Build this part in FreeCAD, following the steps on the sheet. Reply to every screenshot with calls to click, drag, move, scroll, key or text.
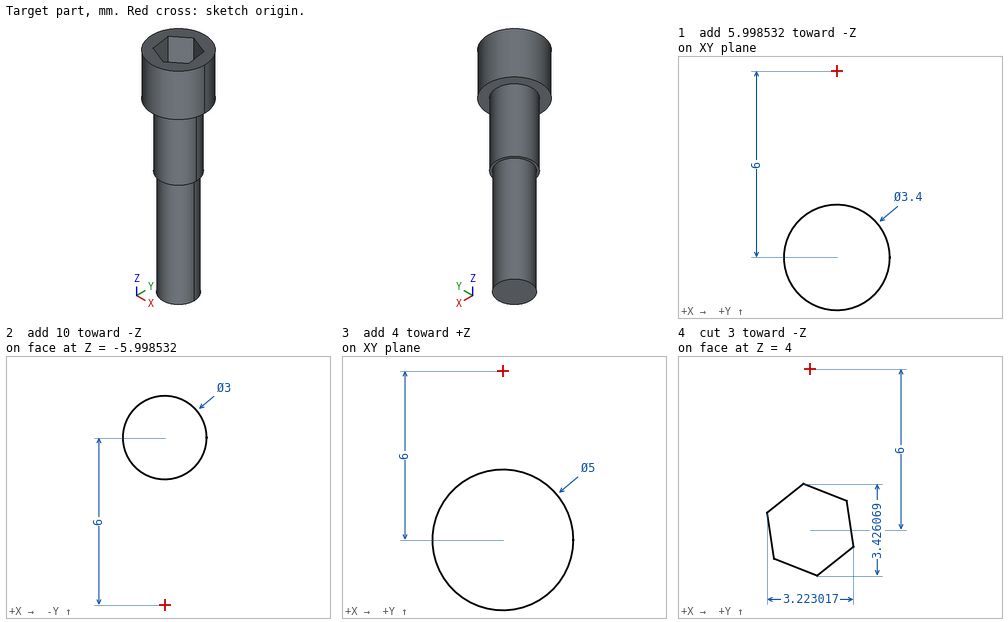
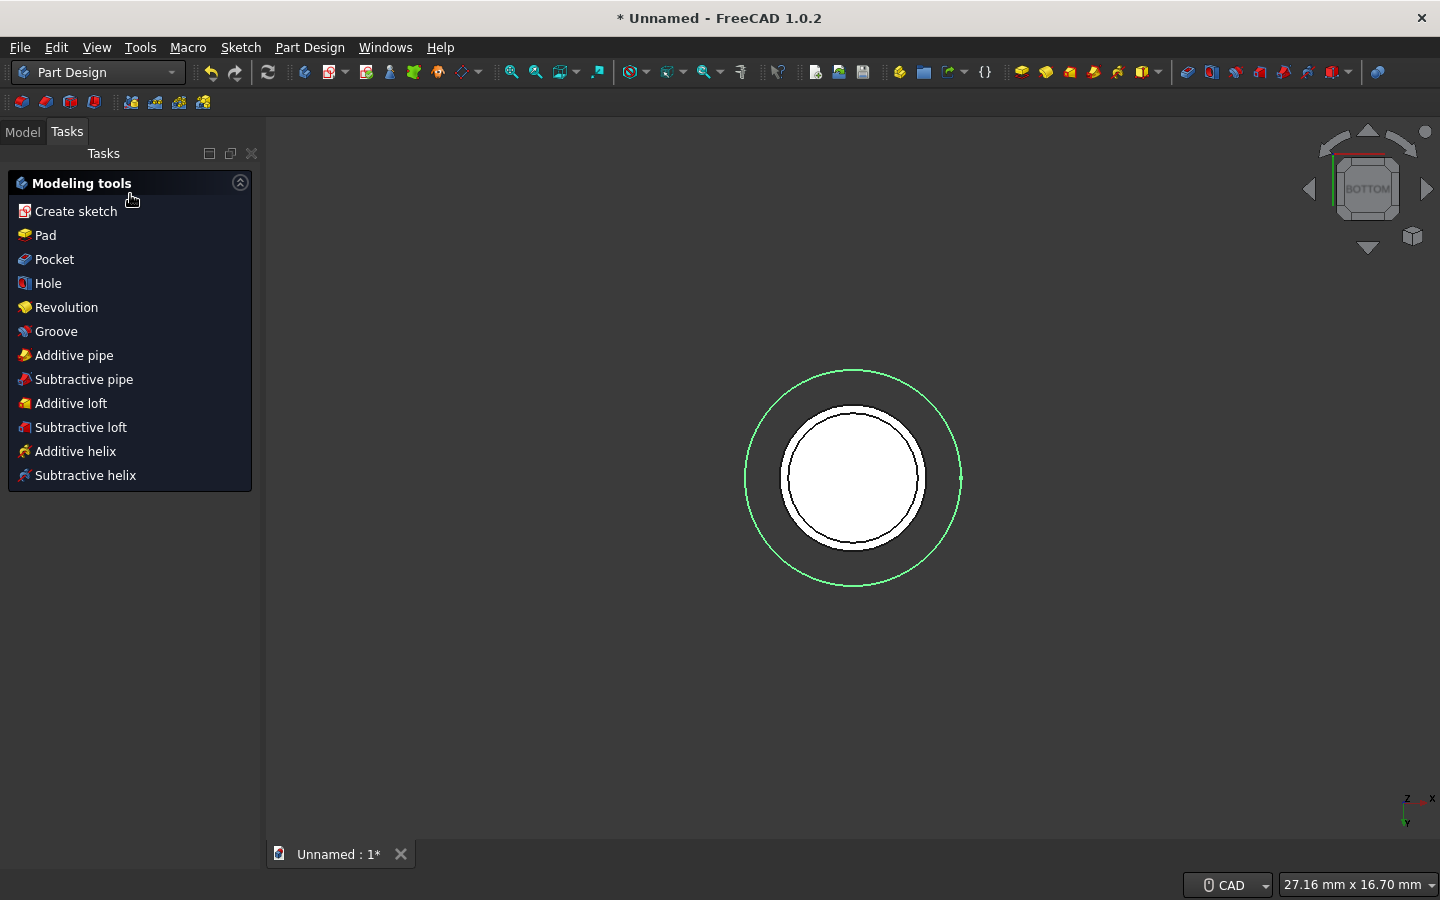
click(1022, 72)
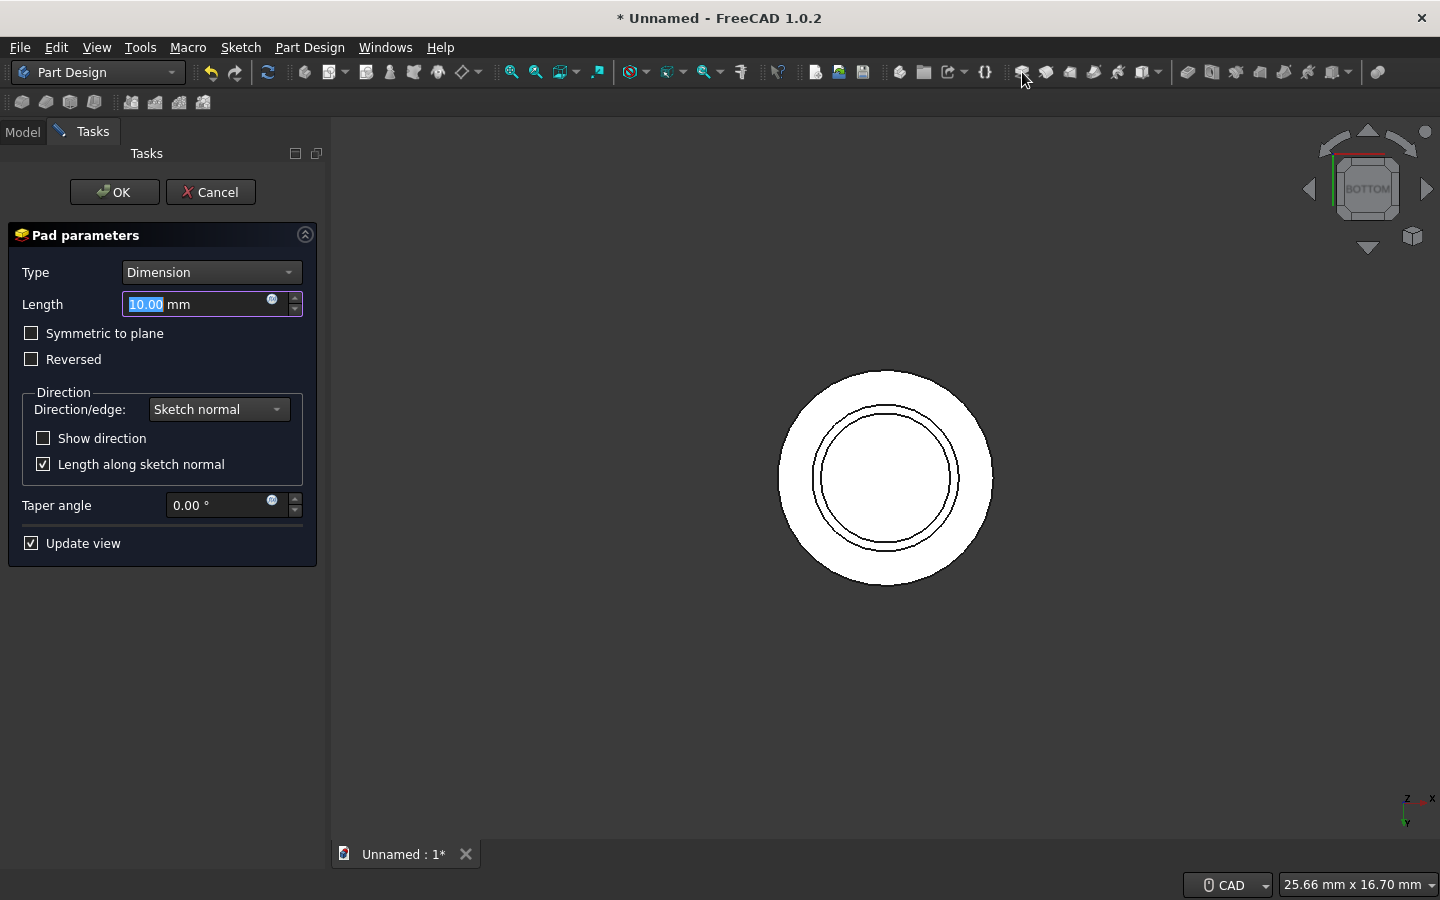
text(4)
key(Tab)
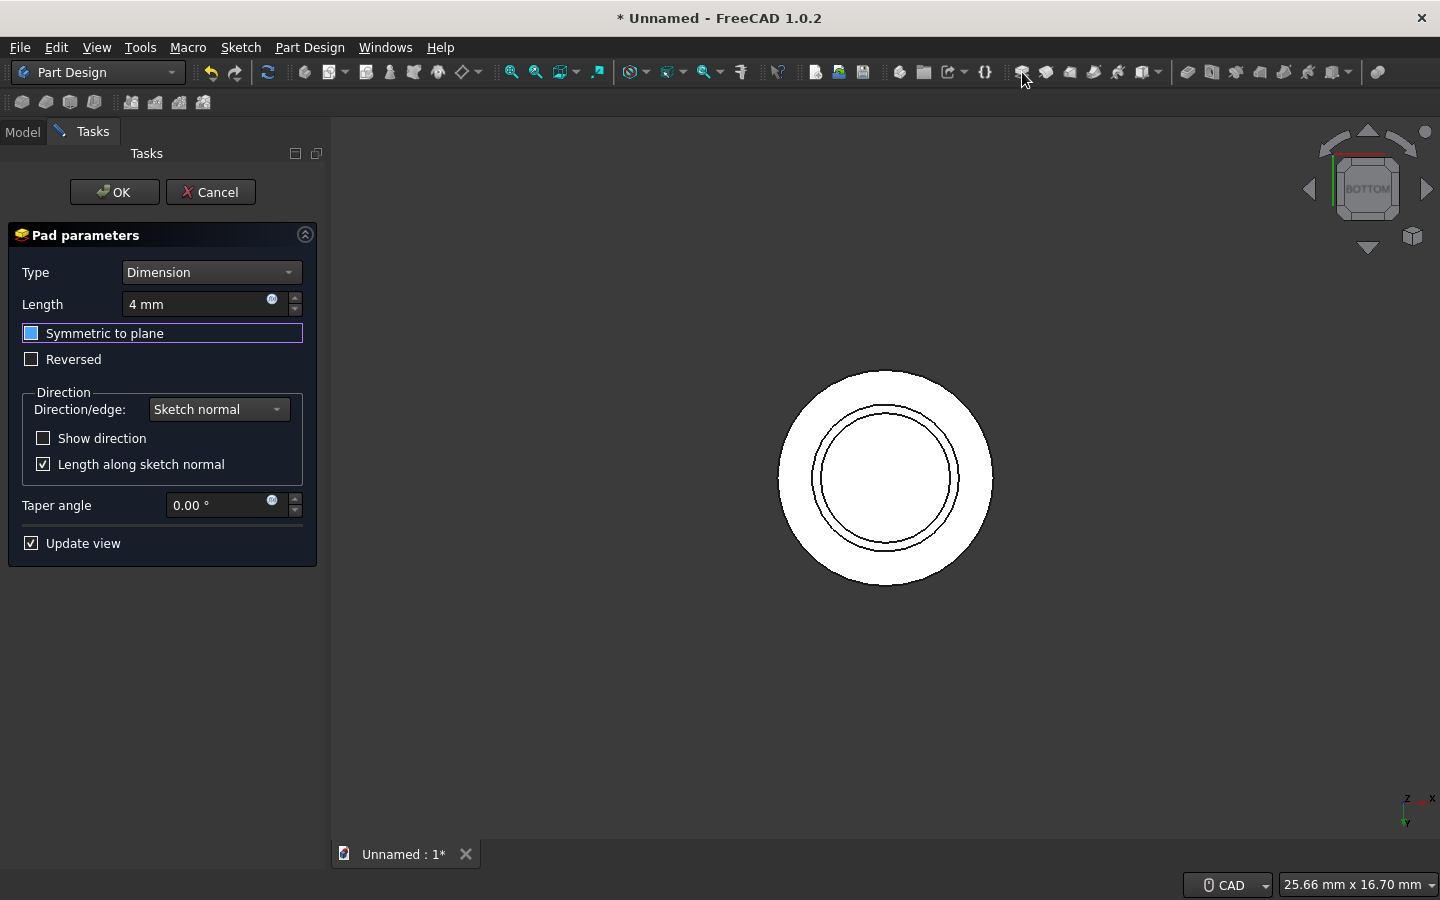
click(115, 192)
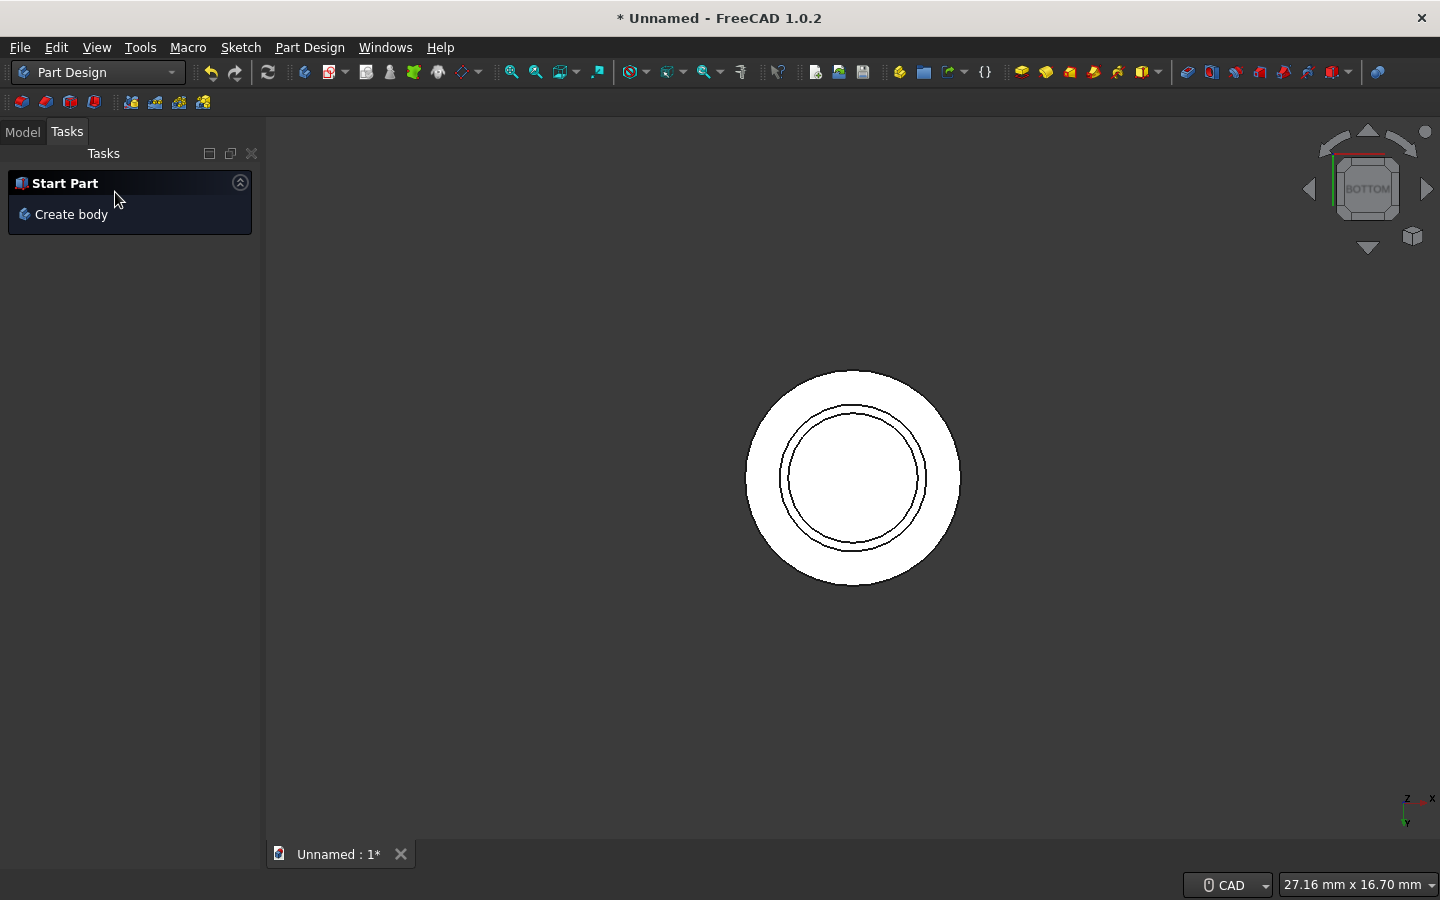
key(v)
key(f)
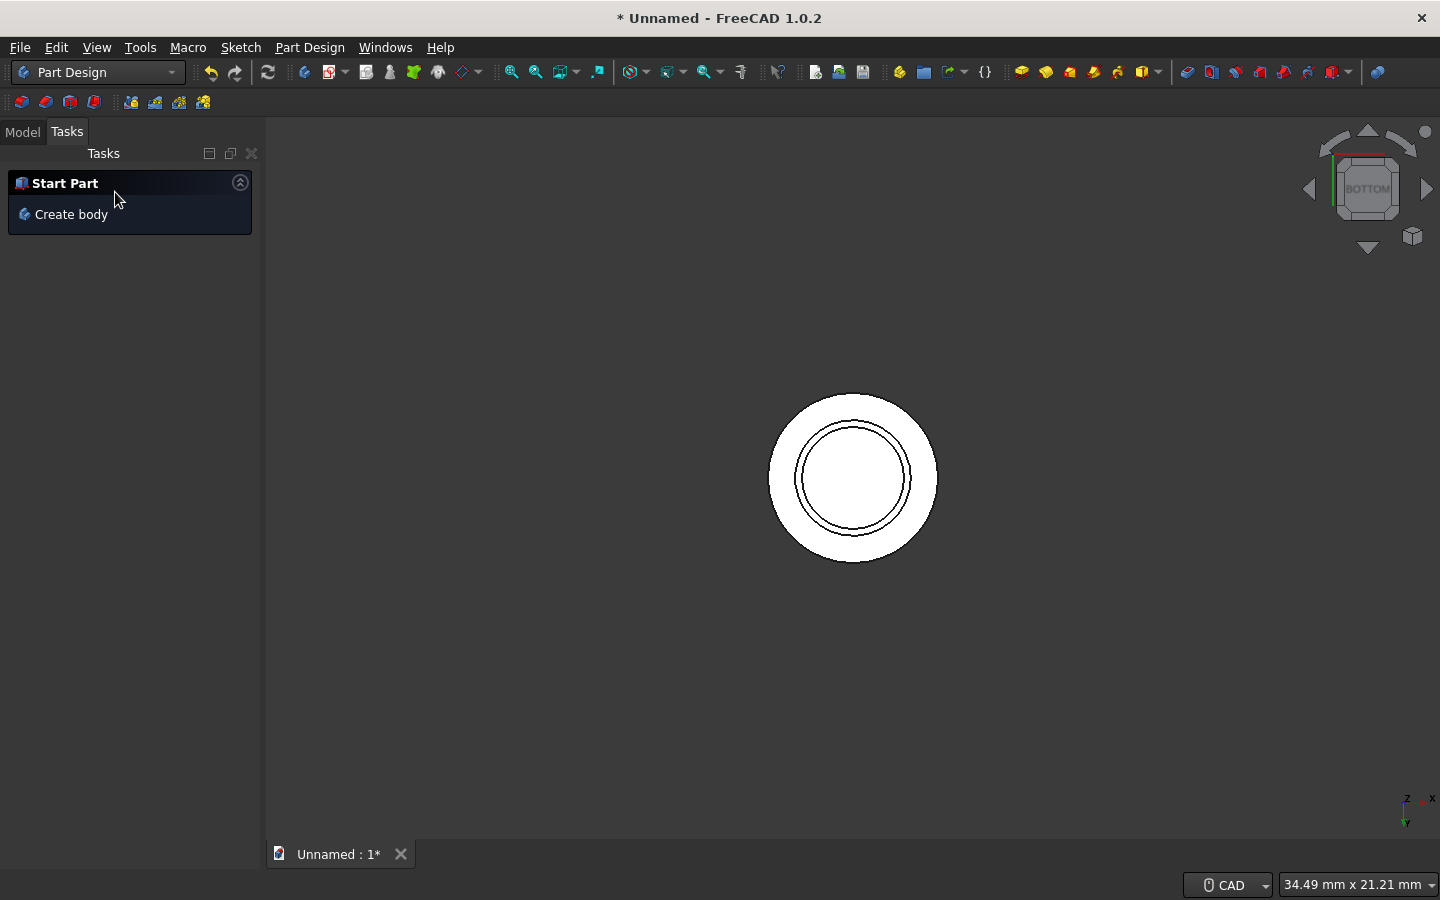
key(0)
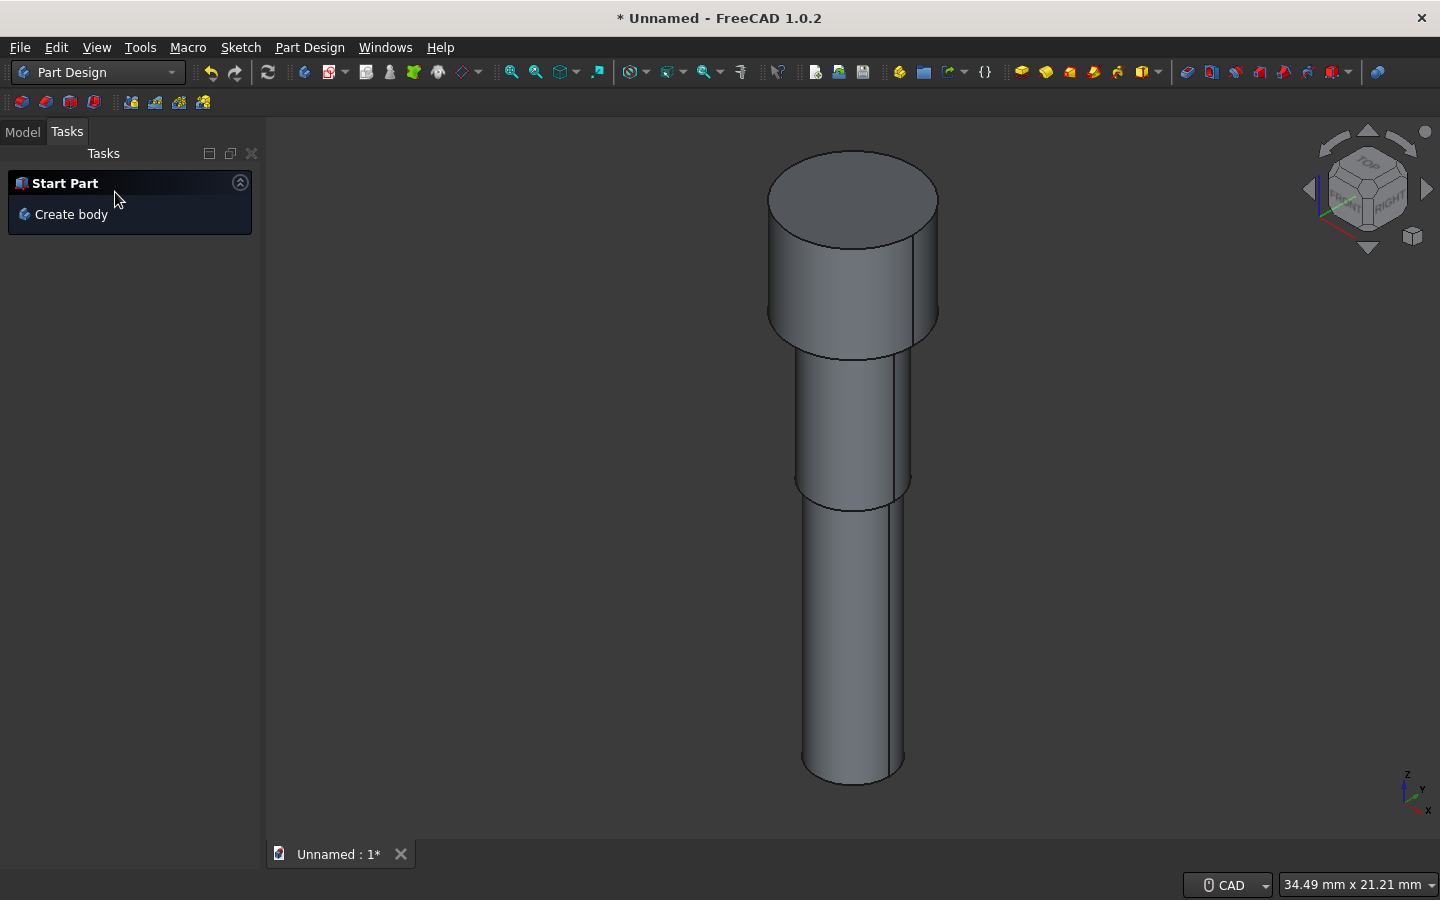
click(853, 199)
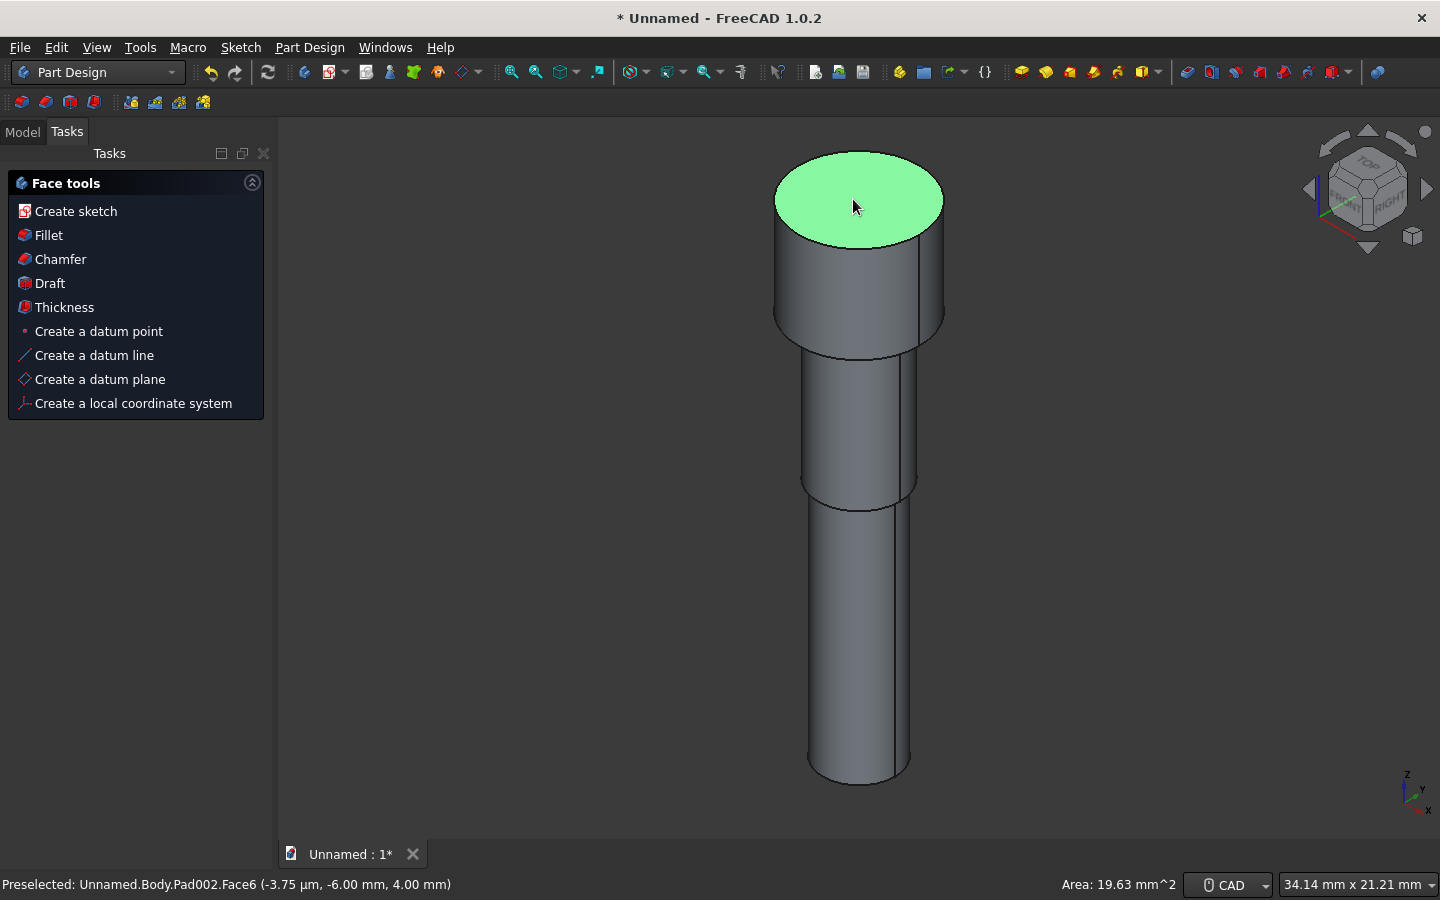
click(330, 72)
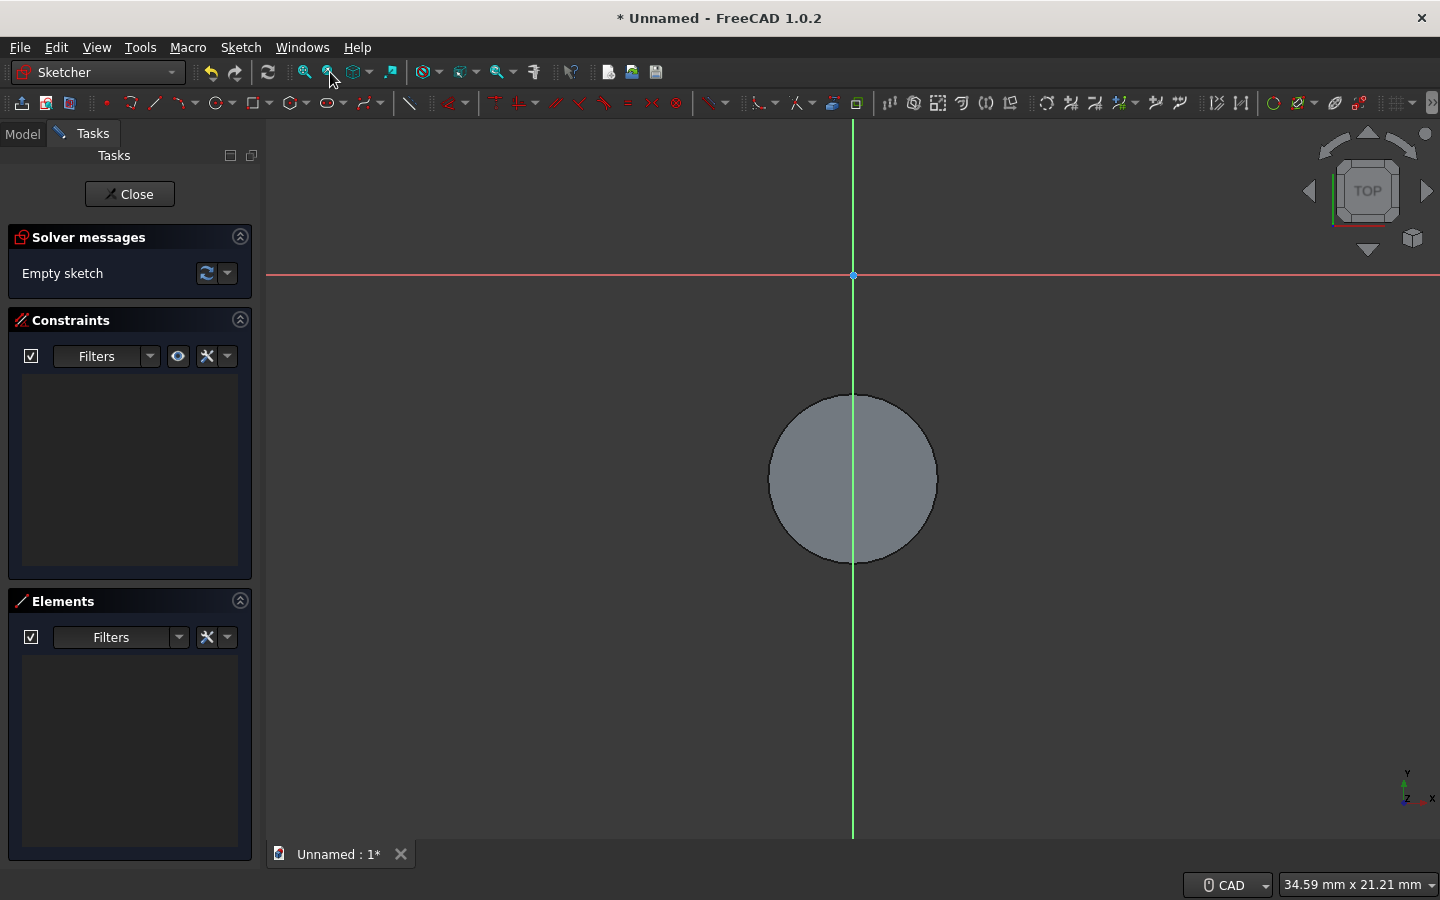
scroll(936, 318, up, 3)